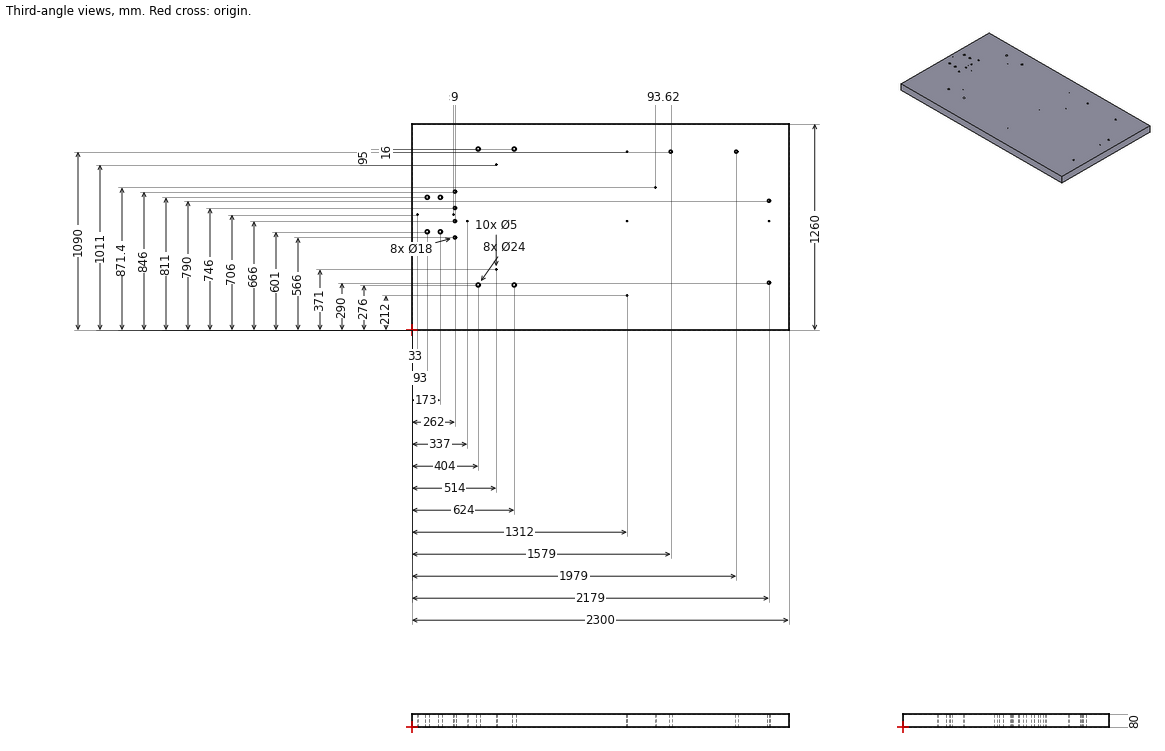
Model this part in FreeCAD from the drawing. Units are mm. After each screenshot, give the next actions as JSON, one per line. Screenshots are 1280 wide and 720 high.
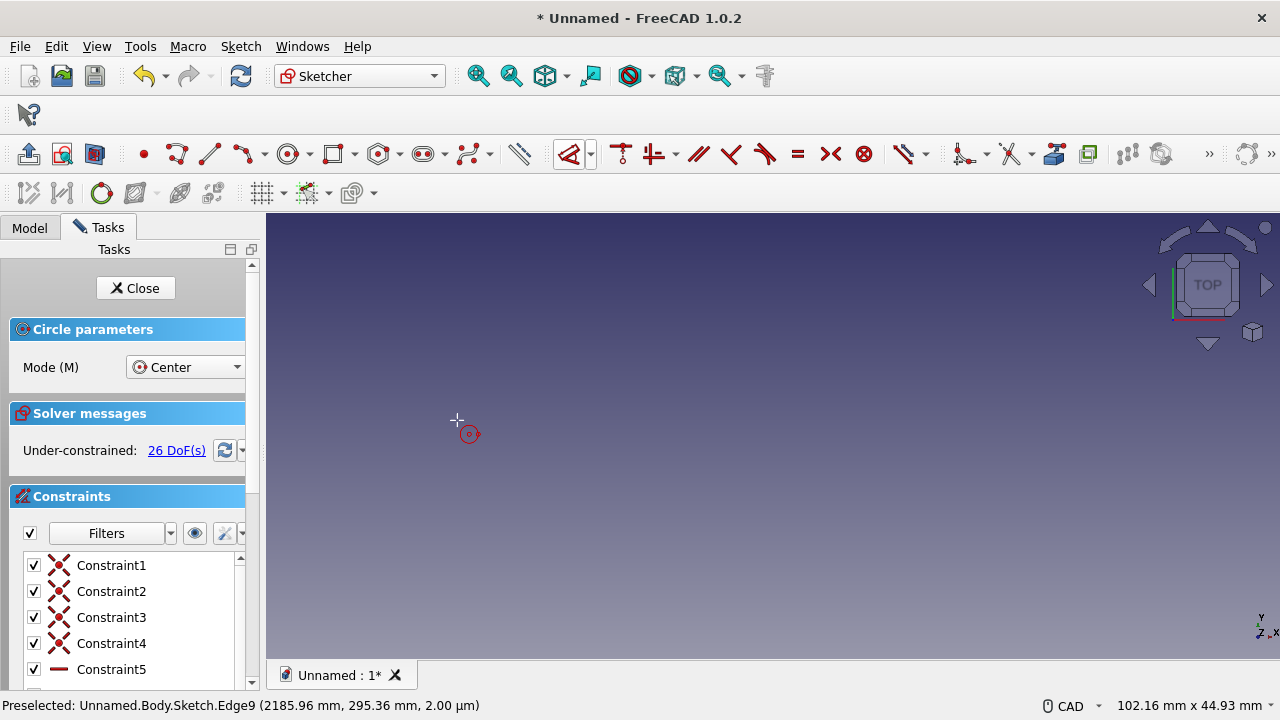
{"action": "scroll", "coordinate": [704, 436], "scroll_direction": "down", "scroll_amount": 15}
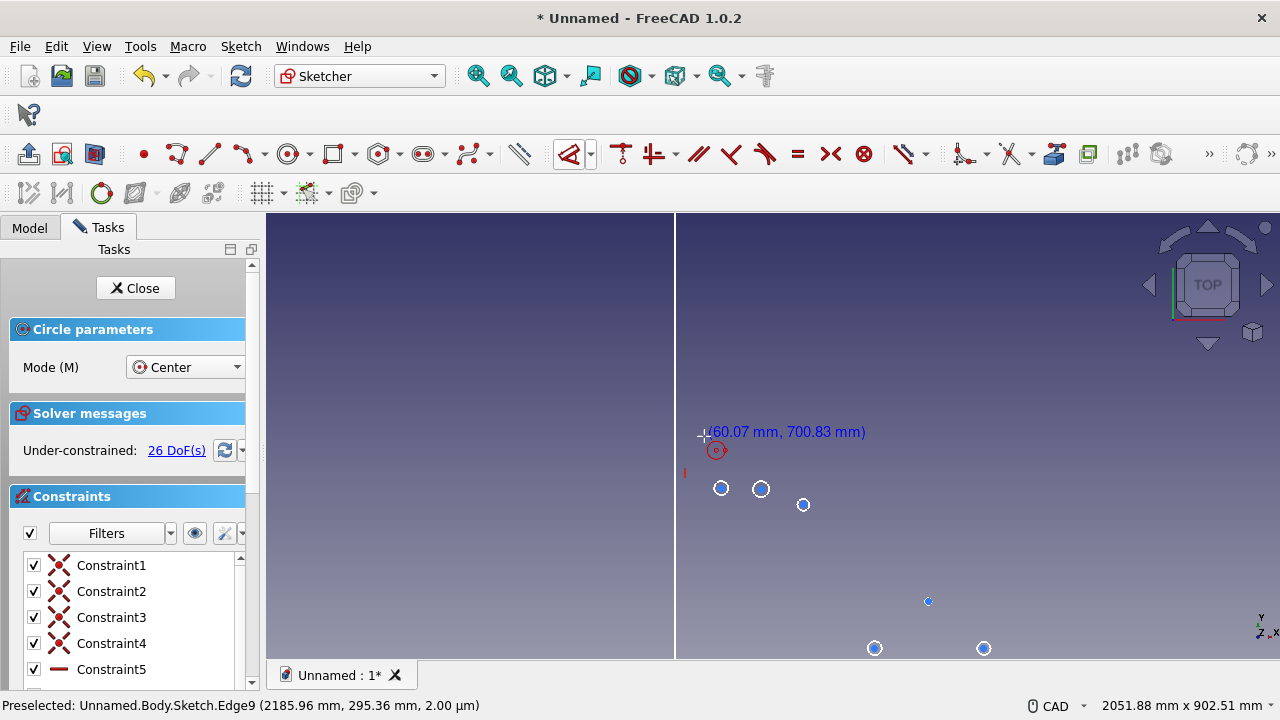
{"action": "scroll", "coordinate": [294, 407], "scroll_direction": "down", "scroll_amount": 4}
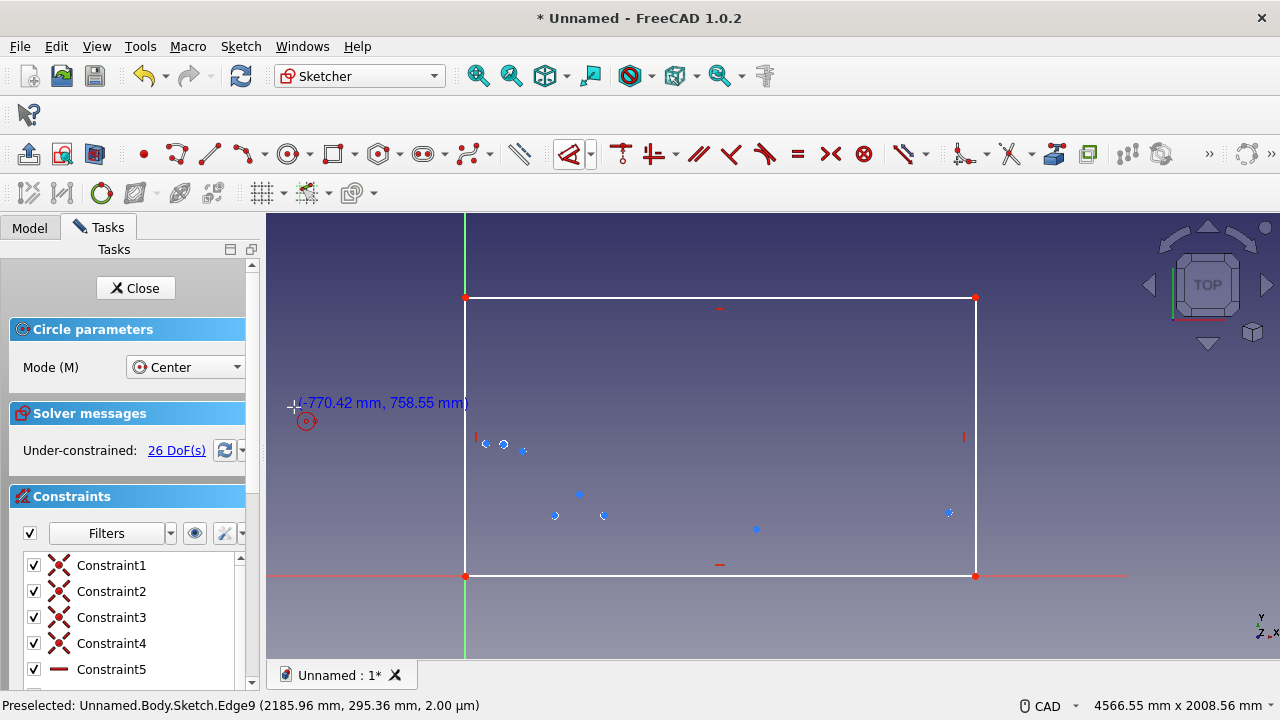
{"action": "scroll", "coordinate": [472, 419], "scroll_direction": "up", "scroll_amount": 4}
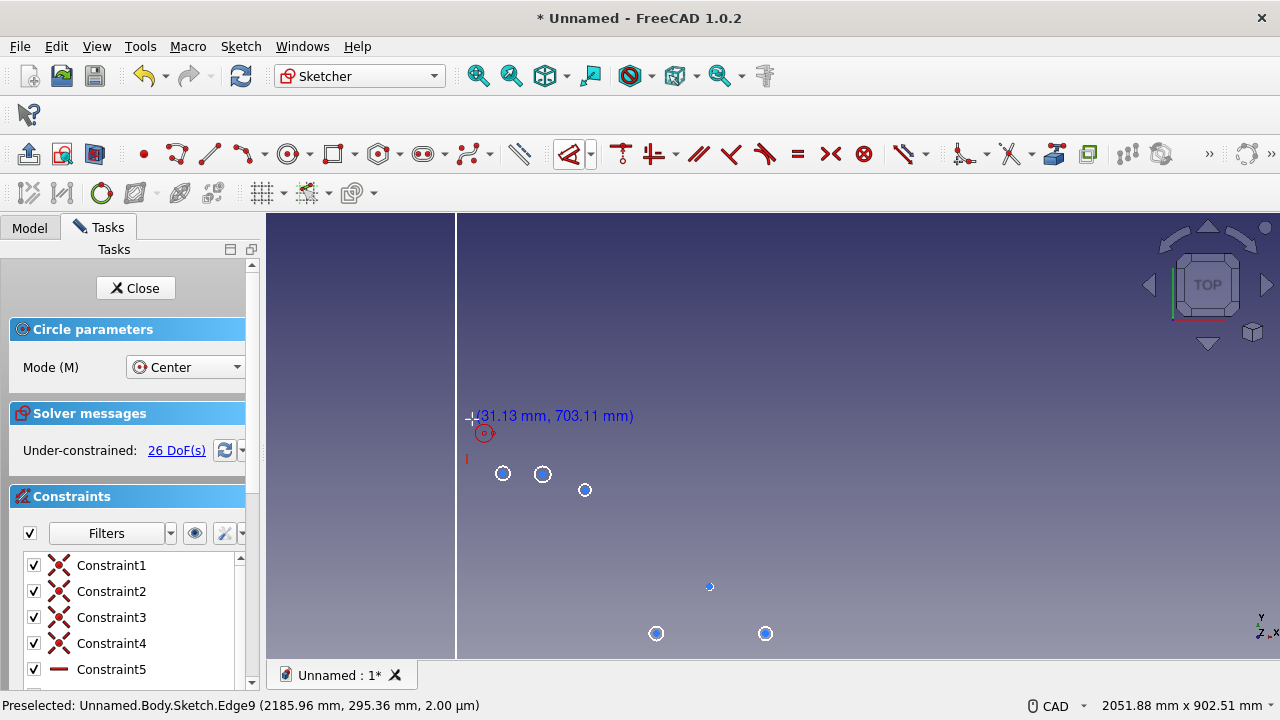
{"action": "left_click", "coordinate": [473, 419]}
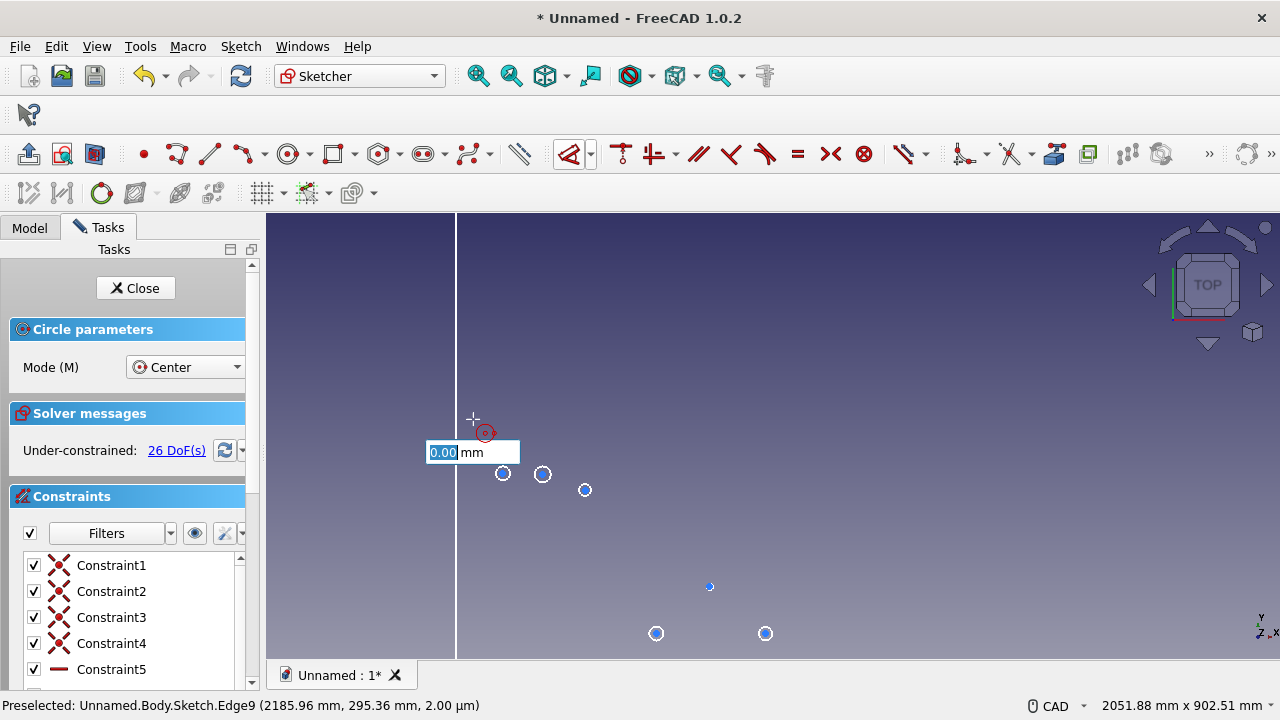
{"action": "scroll", "coordinate": [474, 418], "scroll_direction": "up", "scroll_amount": 13}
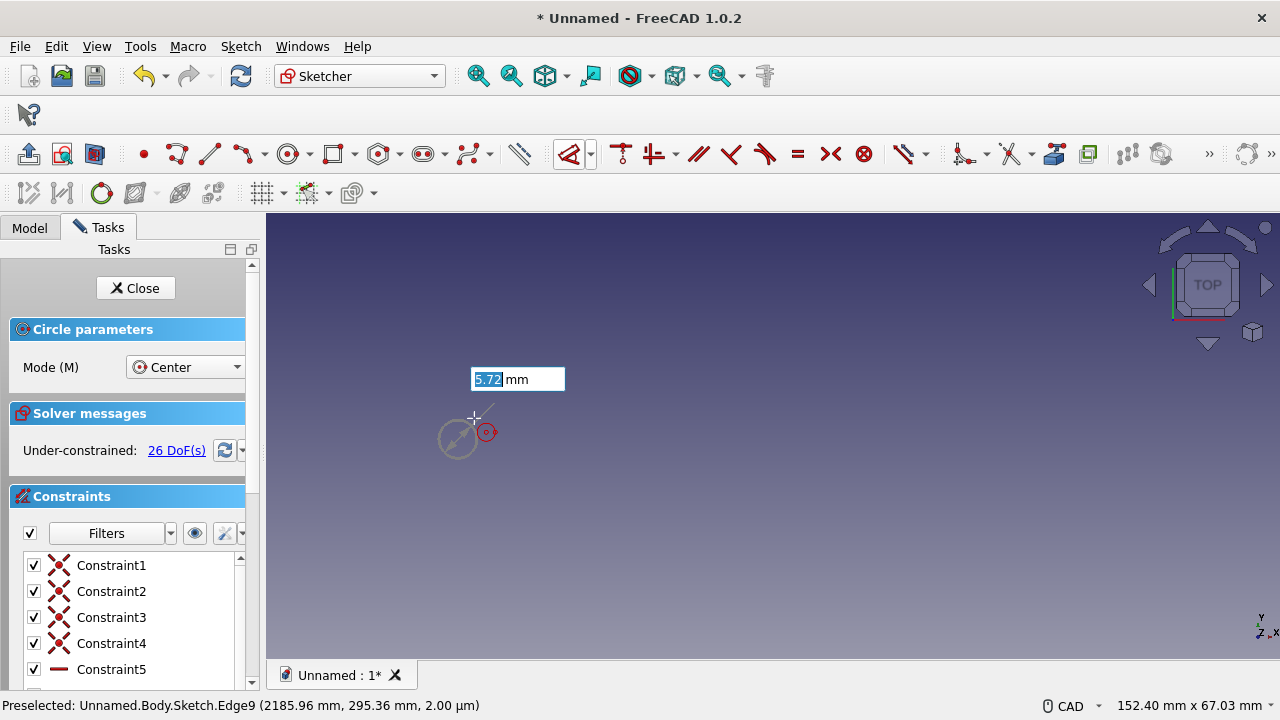
{"action": "left_click", "coordinate": [465, 417]}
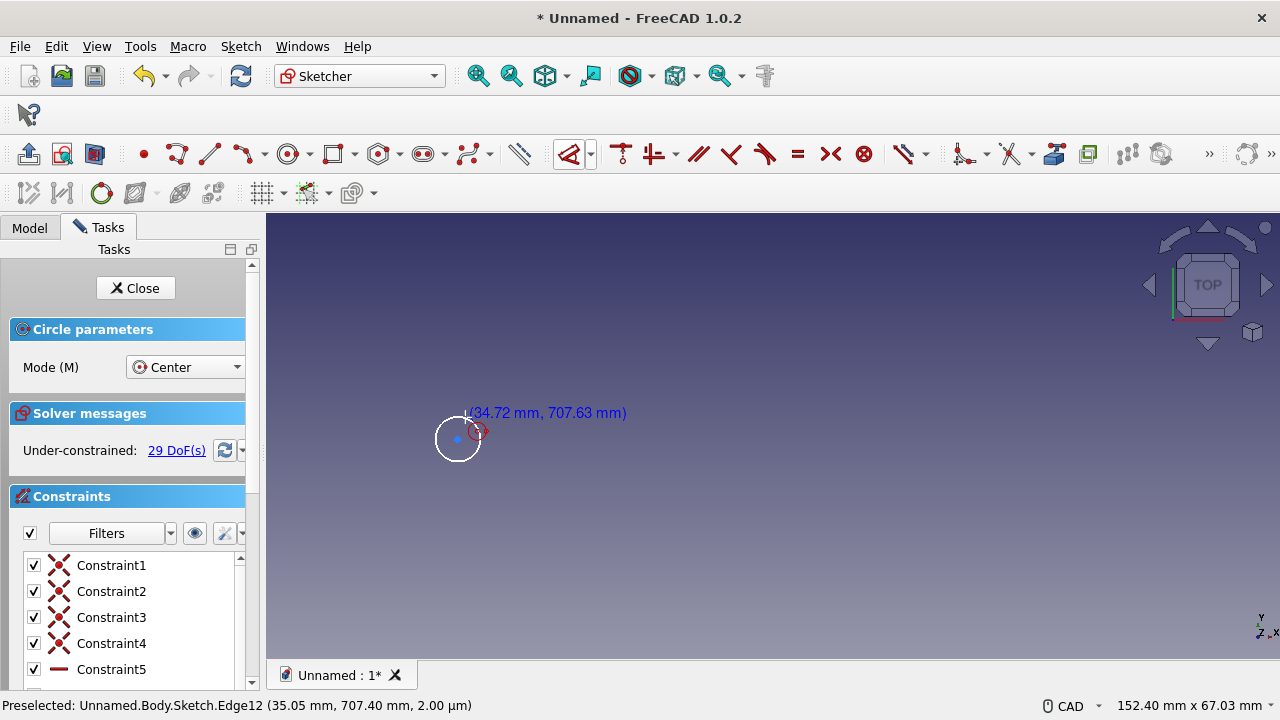
{"action": "scroll", "coordinate": [457, 419], "scroll_direction": "down", "scroll_amount": 17}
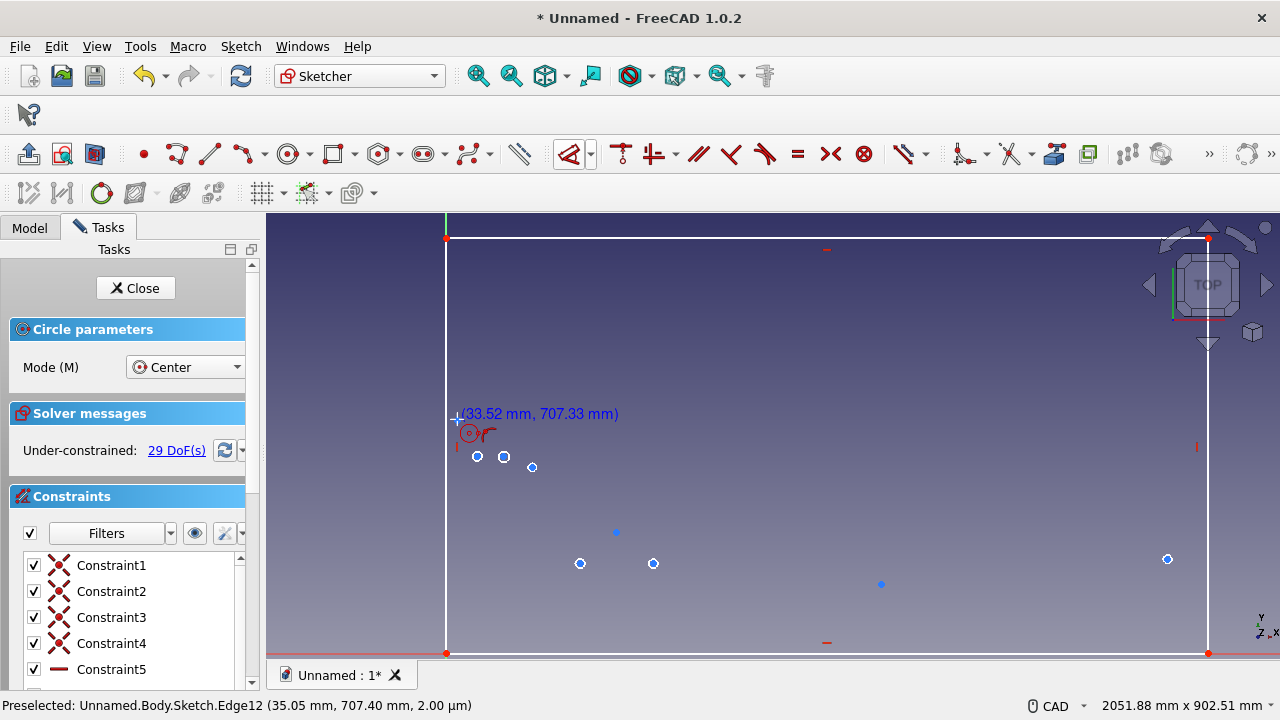
{"action": "scroll", "coordinate": [508, 429], "scroll_direction": "up", "scroll_amount": 13}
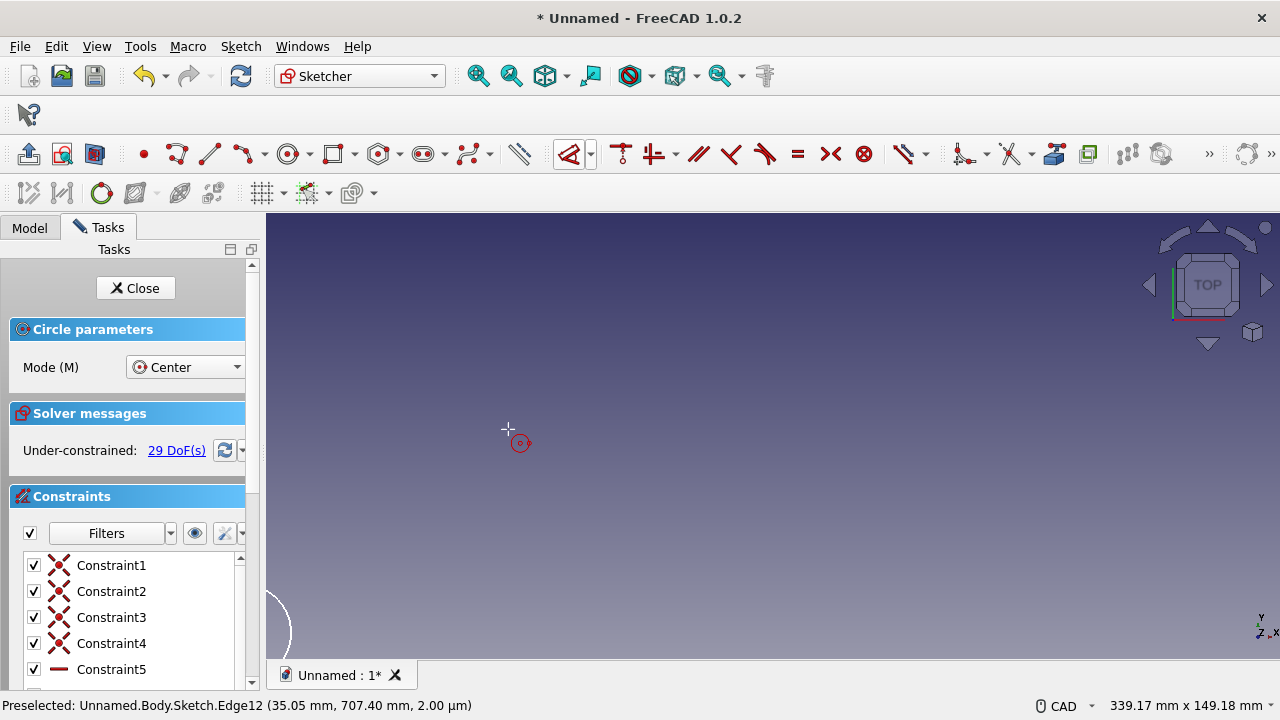
{"action": "scroll", "coordinate": [508, 429], "scroll_direction": "down", "scroll_amount": 13}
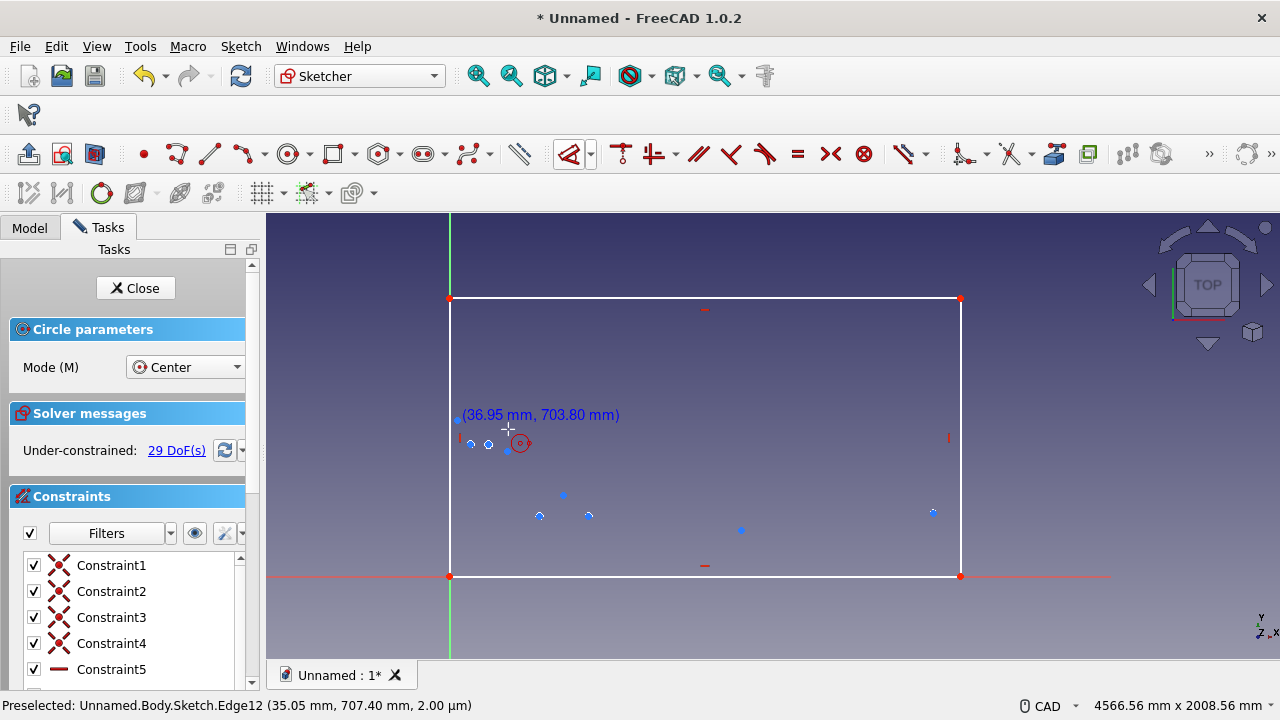
{"action": "left_click", "coordinate": [508, 429]}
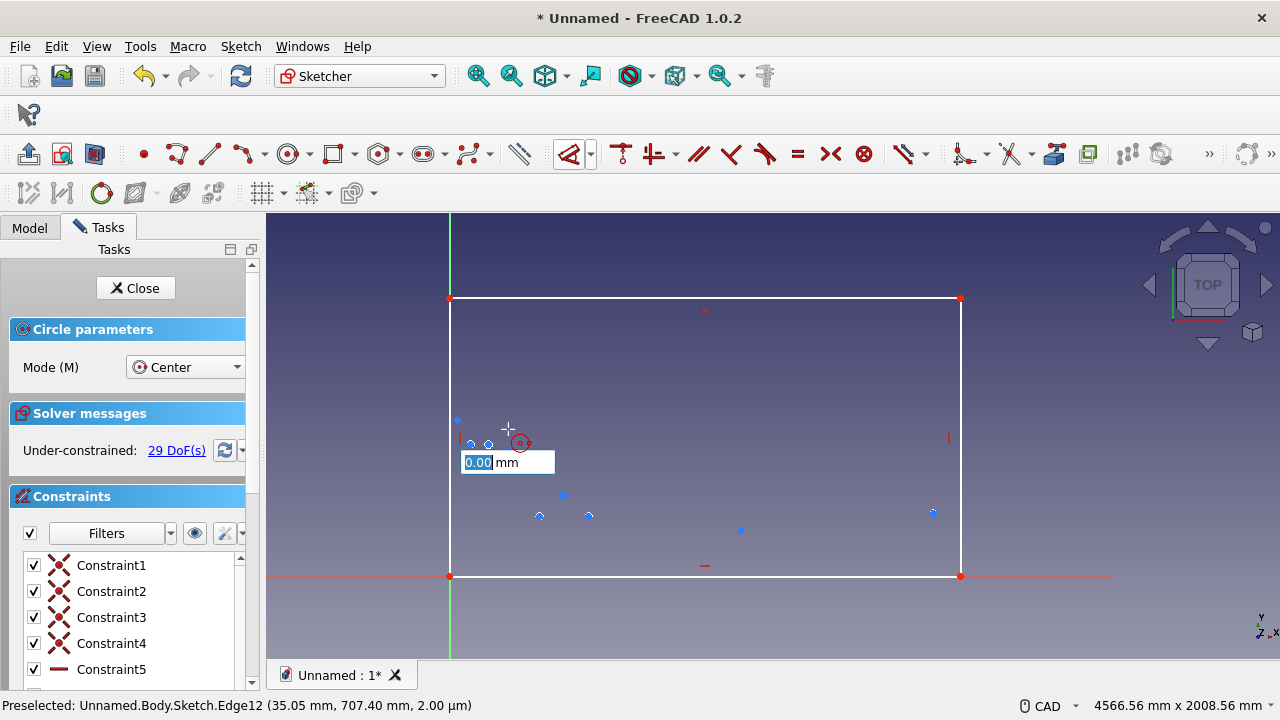
{"action": "scroll", "coordinate": [509, 427], "scroll_direction": "up", "scroll_amount": 11}